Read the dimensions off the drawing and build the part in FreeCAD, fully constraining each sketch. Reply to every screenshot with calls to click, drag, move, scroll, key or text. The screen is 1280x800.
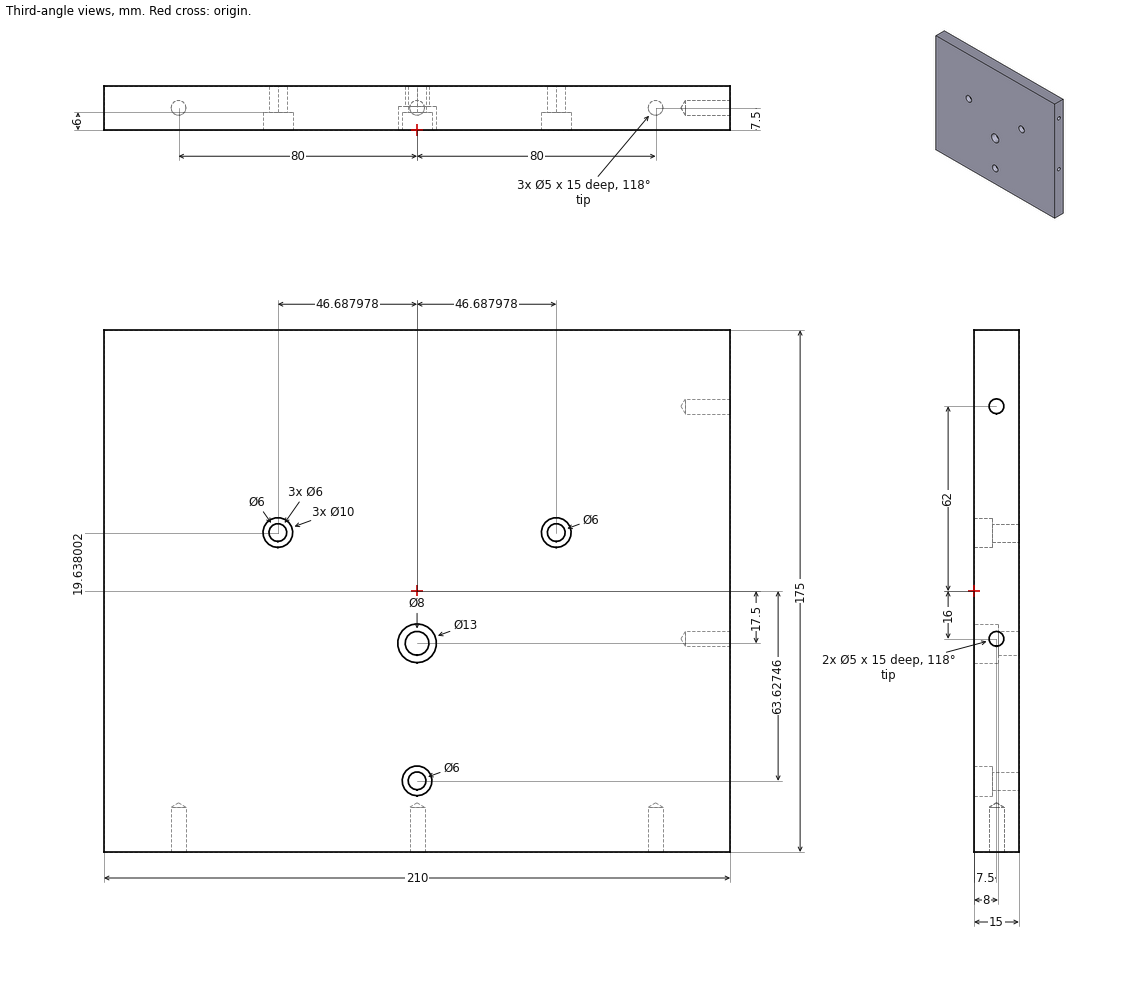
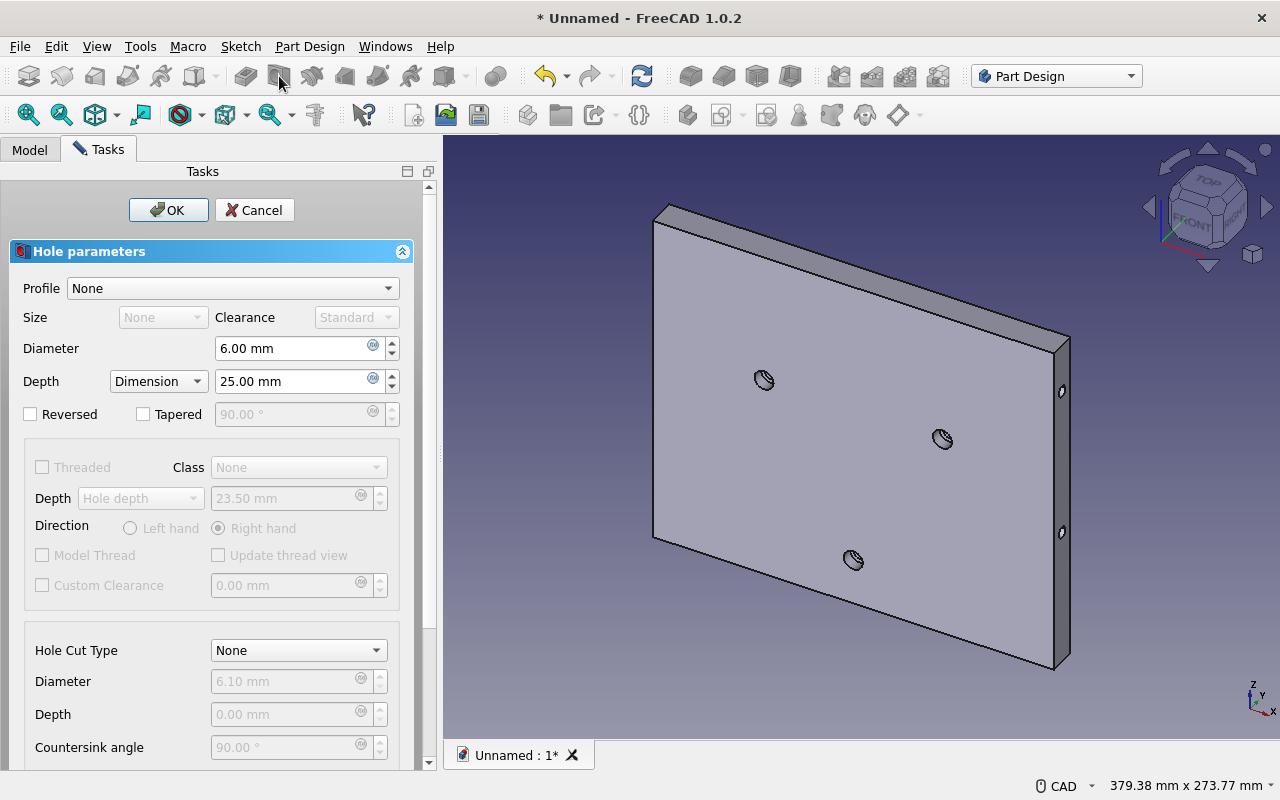
triple_click(300, 348)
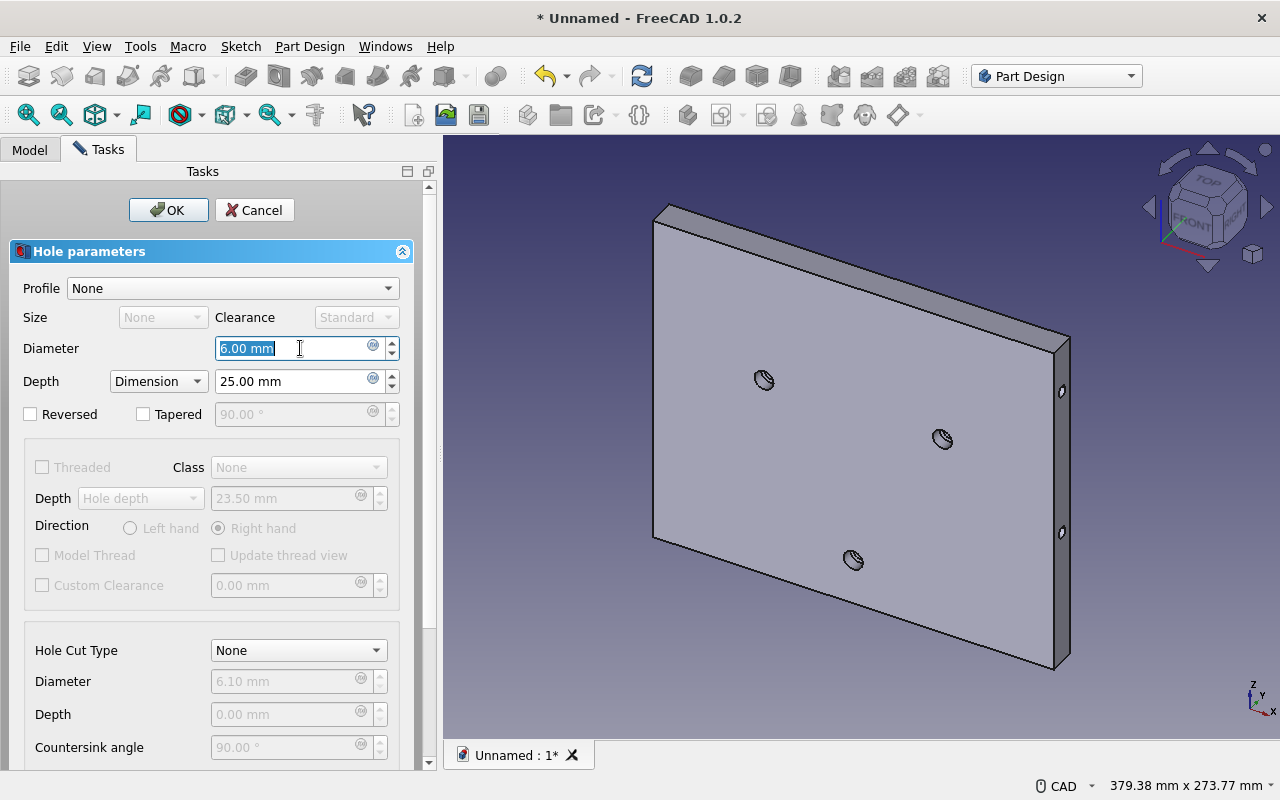
text(5)
key(Tab)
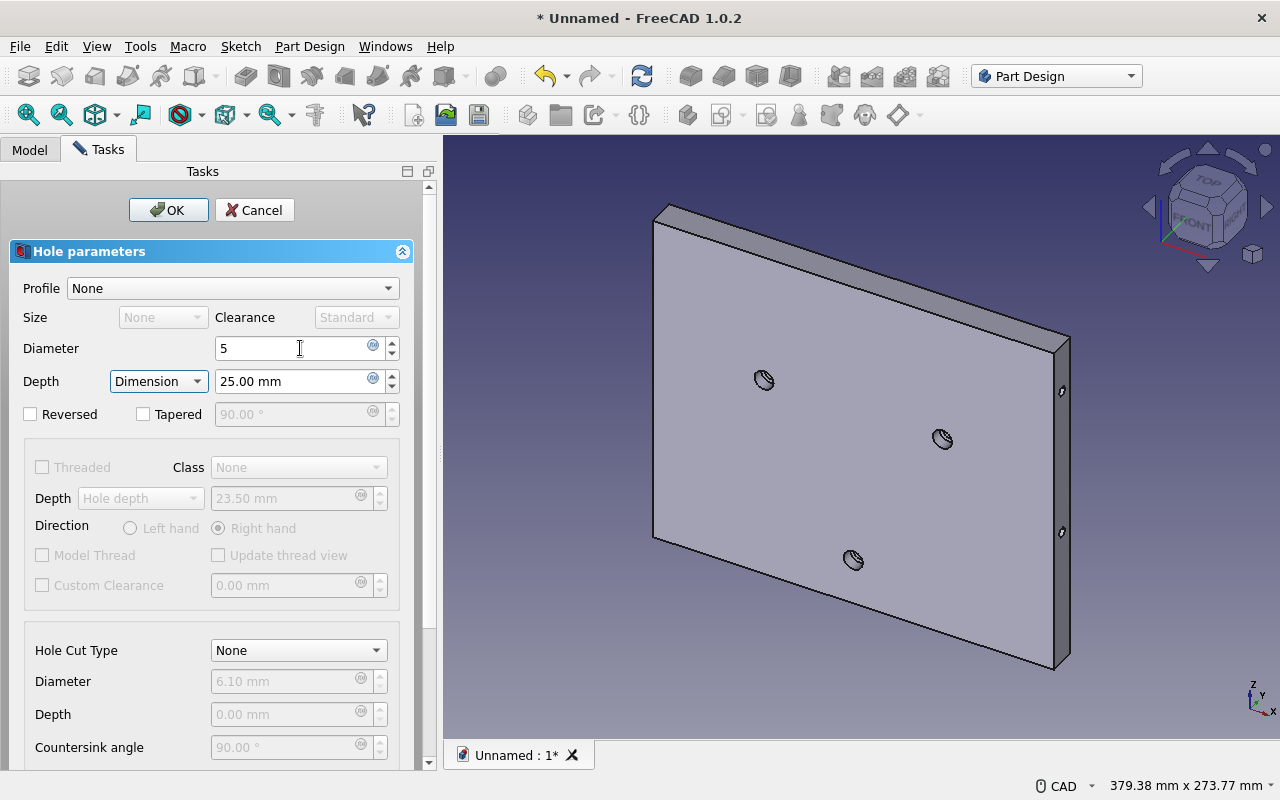
triple_click(300, 382)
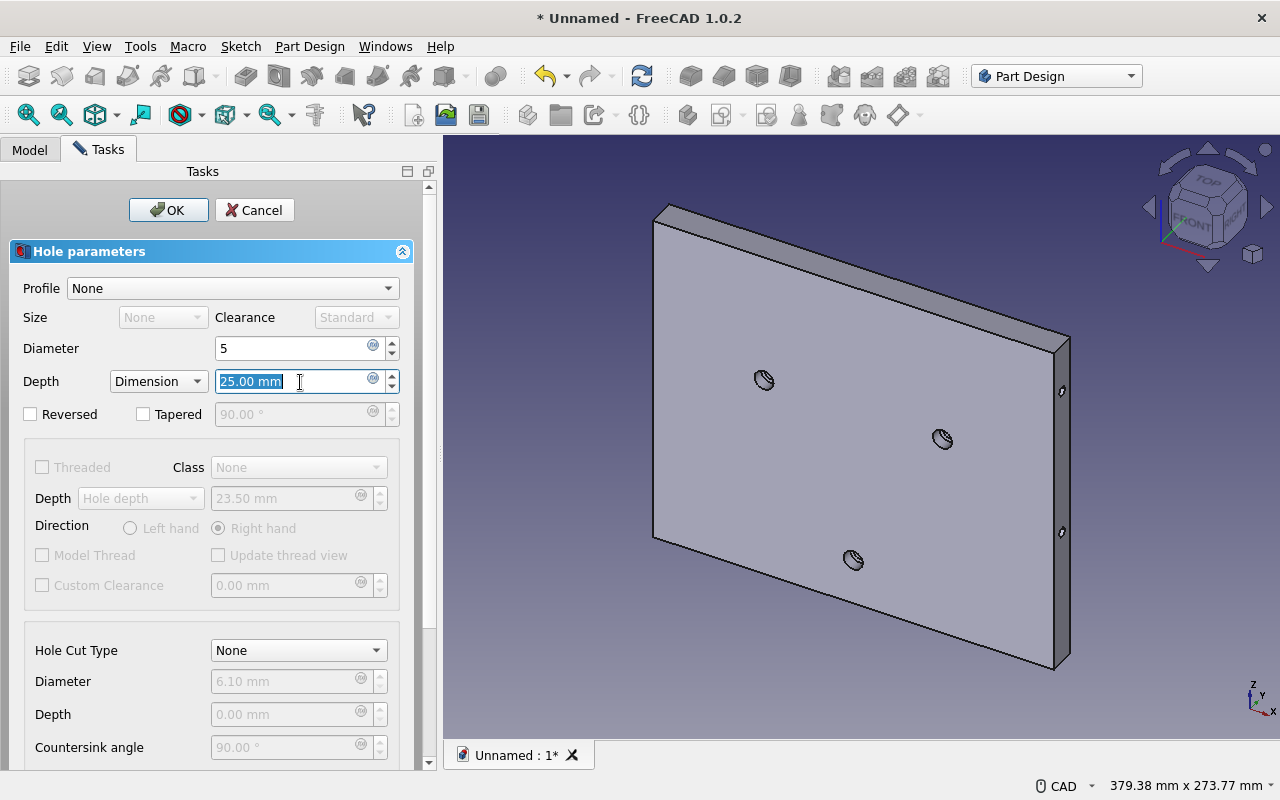
text(15)
key(Tab)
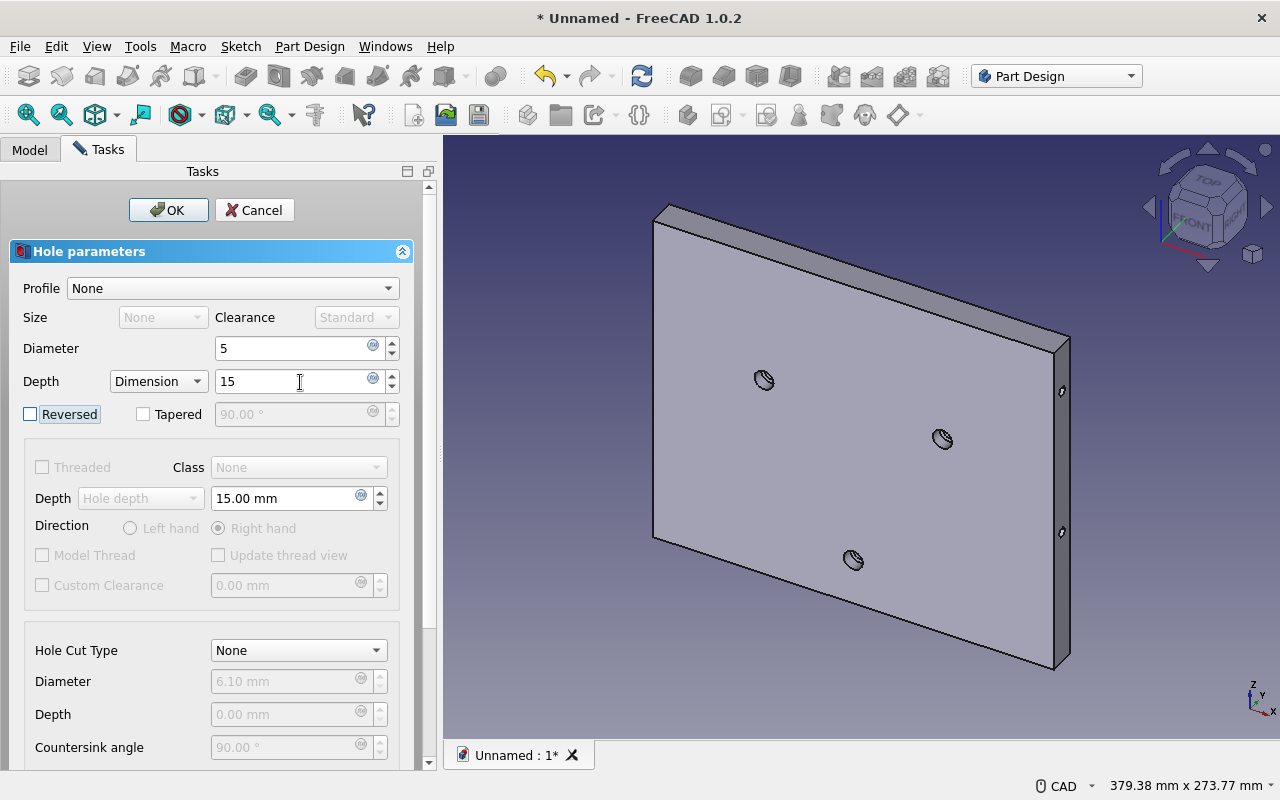
click(169, 210)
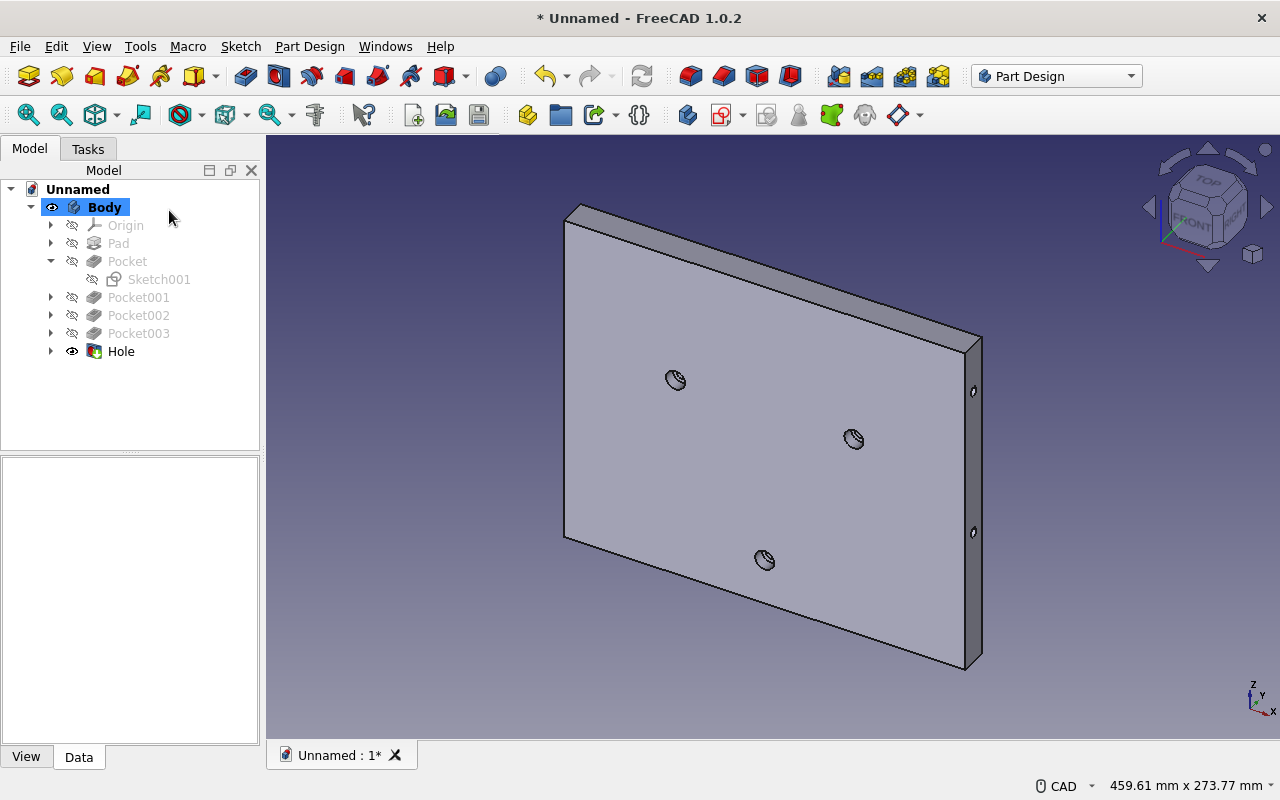
key(5)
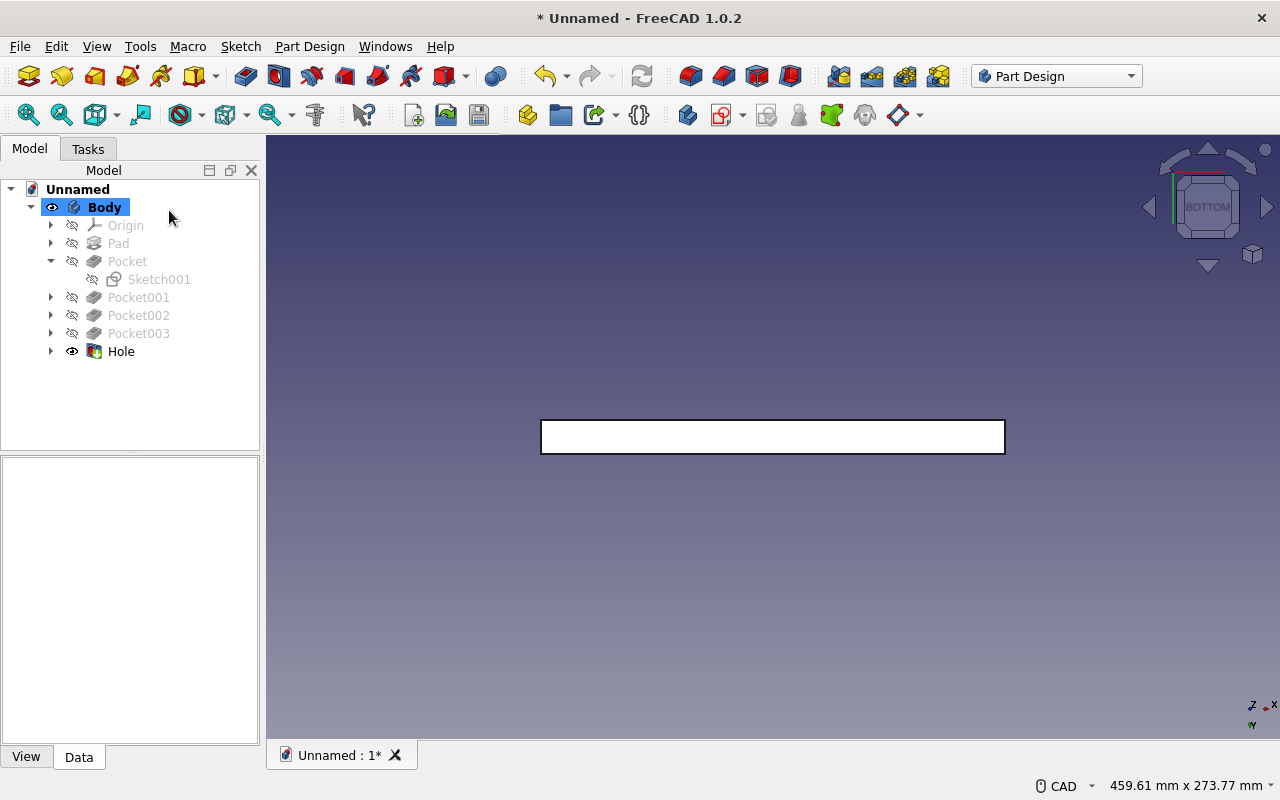
click(972, 436)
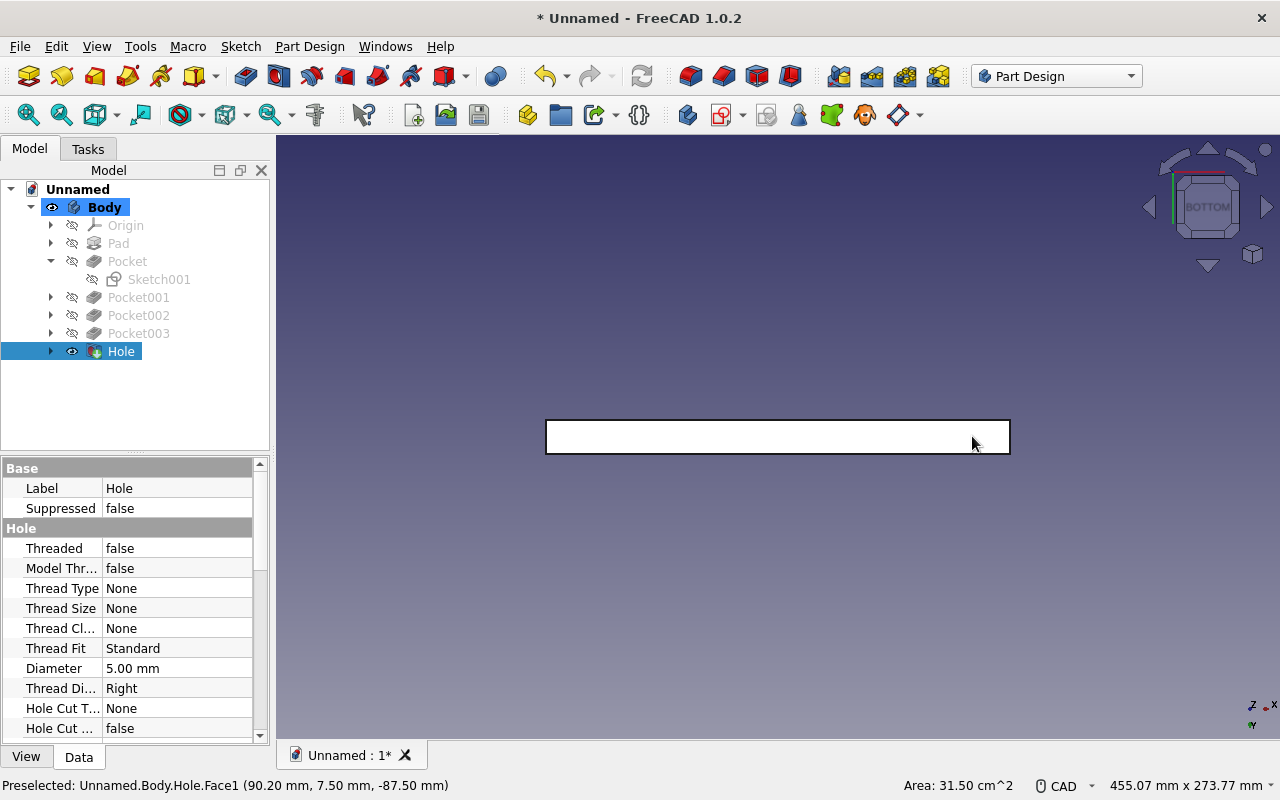
click(720, 116)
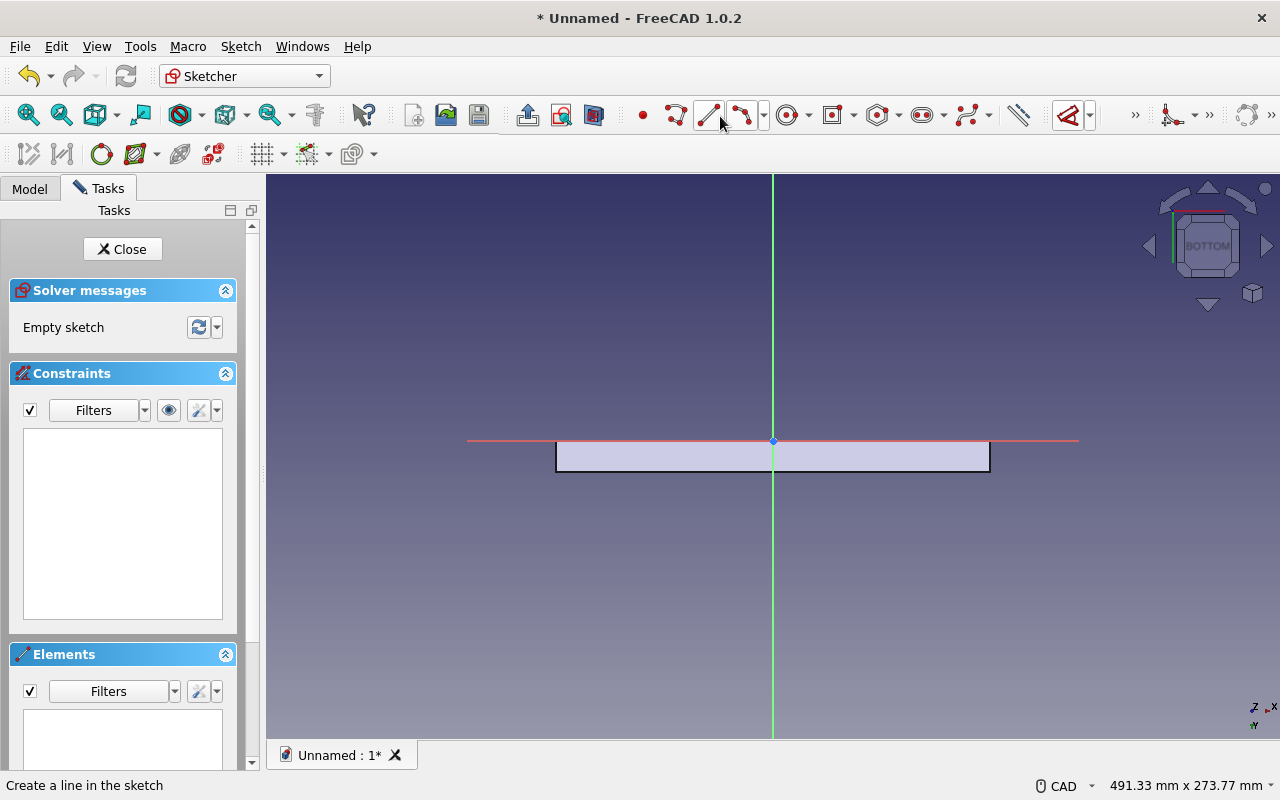
scroll(856, 445, up, 3)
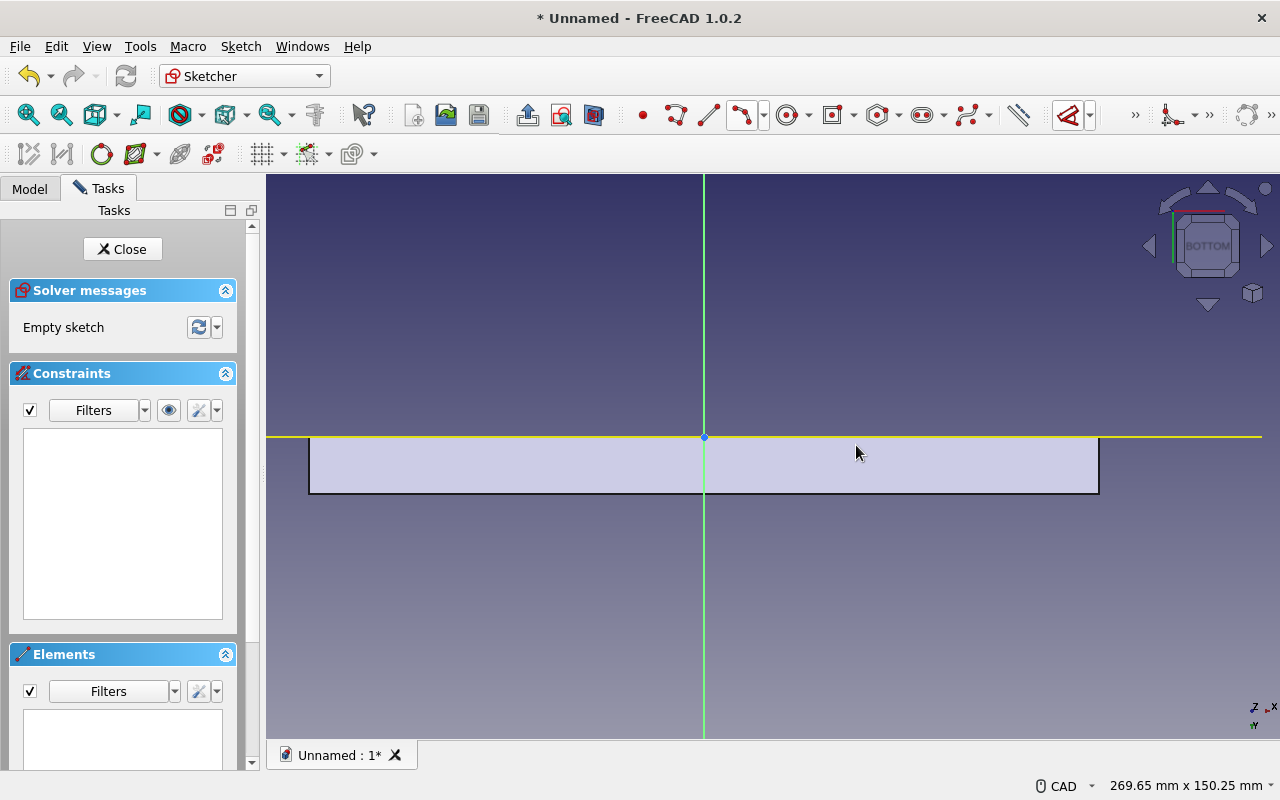
click(786, 116)